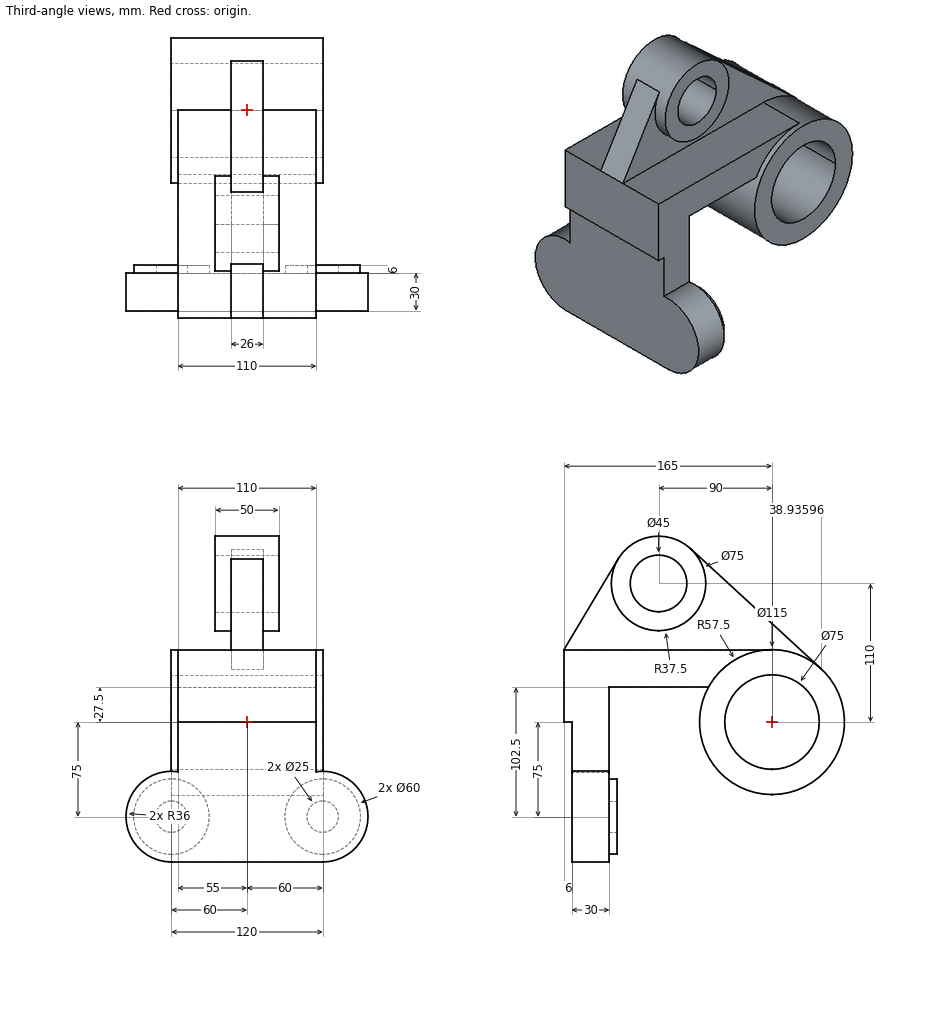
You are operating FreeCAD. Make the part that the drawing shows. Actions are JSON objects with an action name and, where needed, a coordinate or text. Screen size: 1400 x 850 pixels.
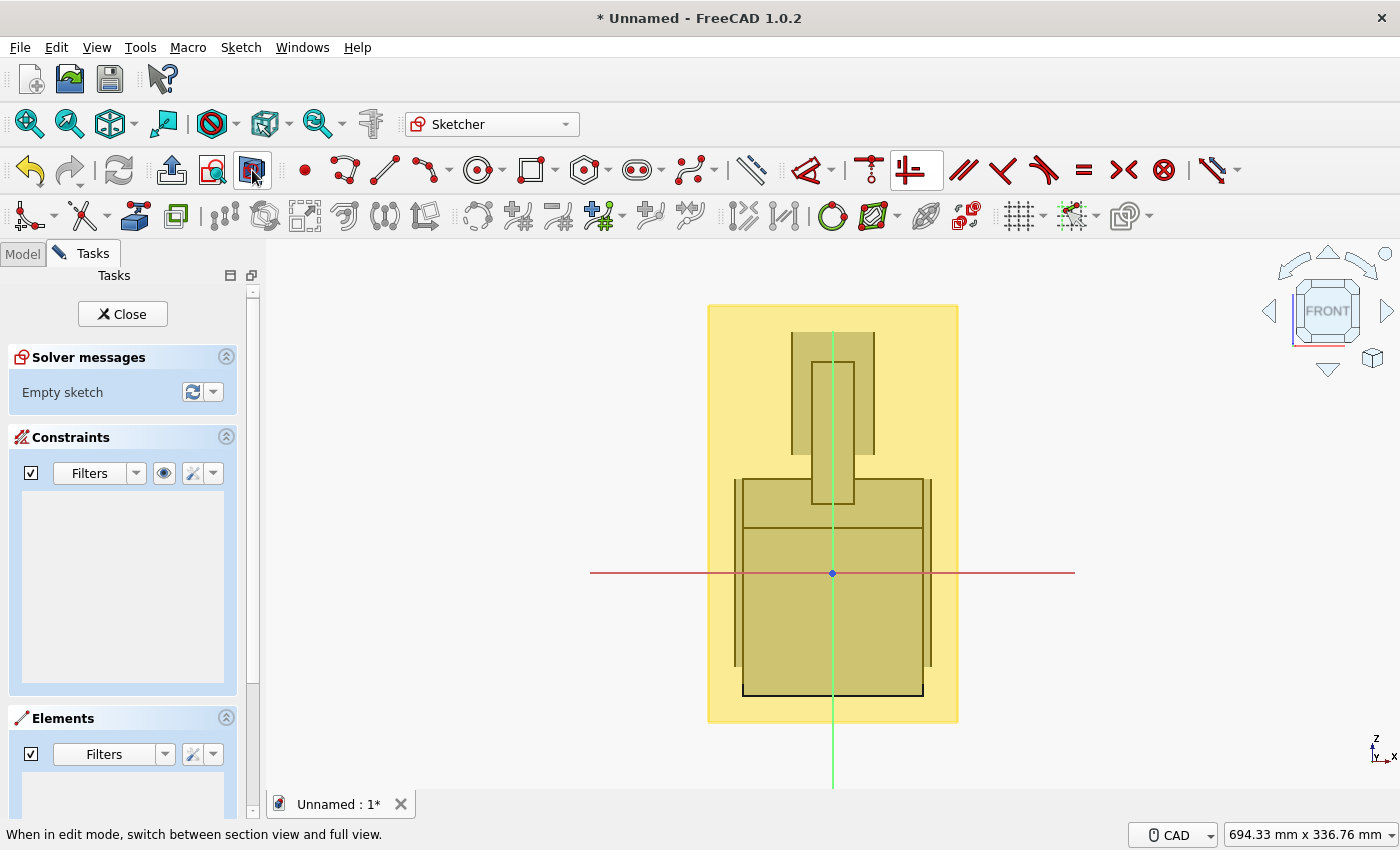
{"action": "scroll", "coordinate": [455, 267], "scroll_direction": "down", "scroll_amount": 1}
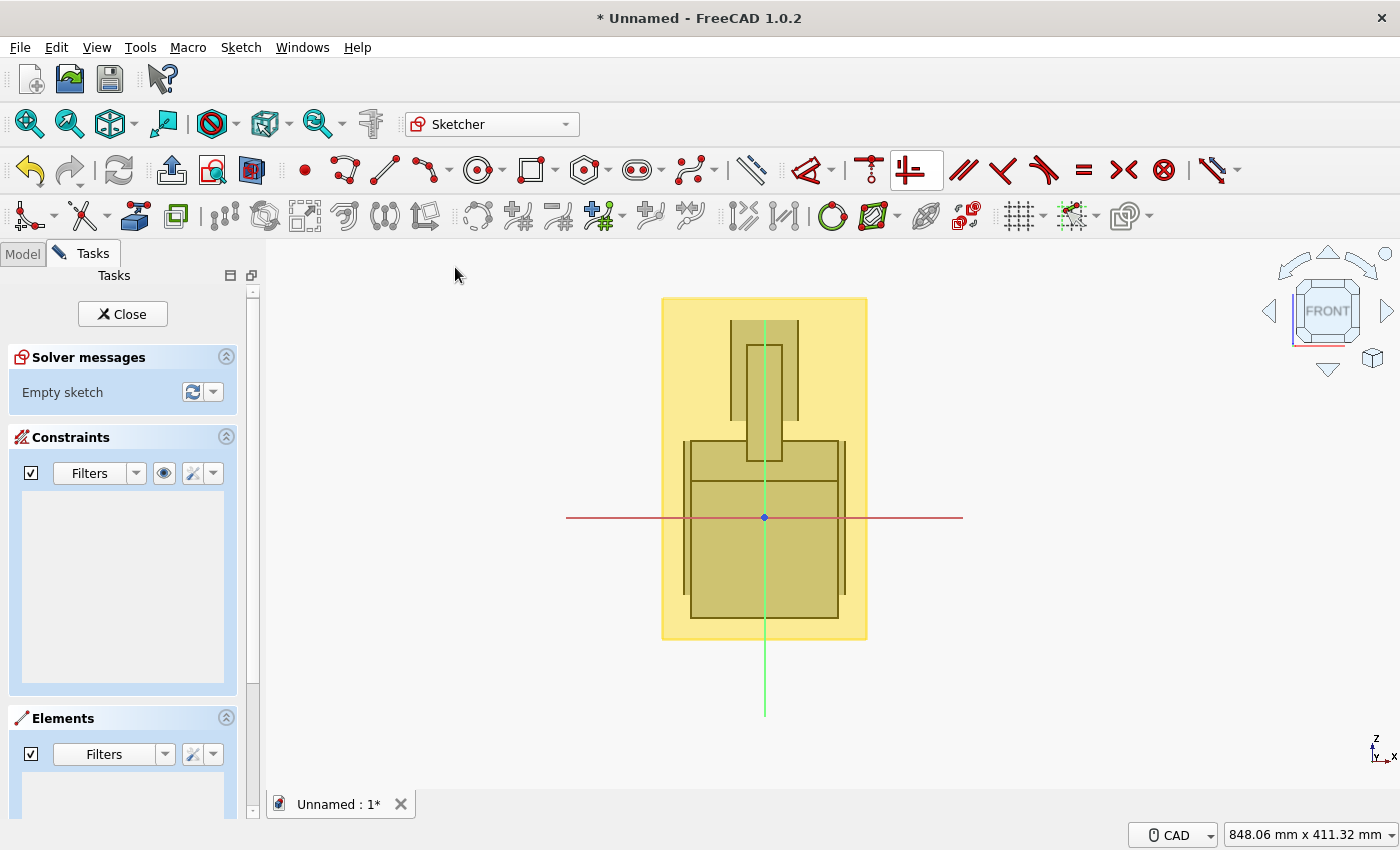
{"action": "scroll", "coordinate": [765, 646], "scroll_direction": "up", "scroll_amount": 3}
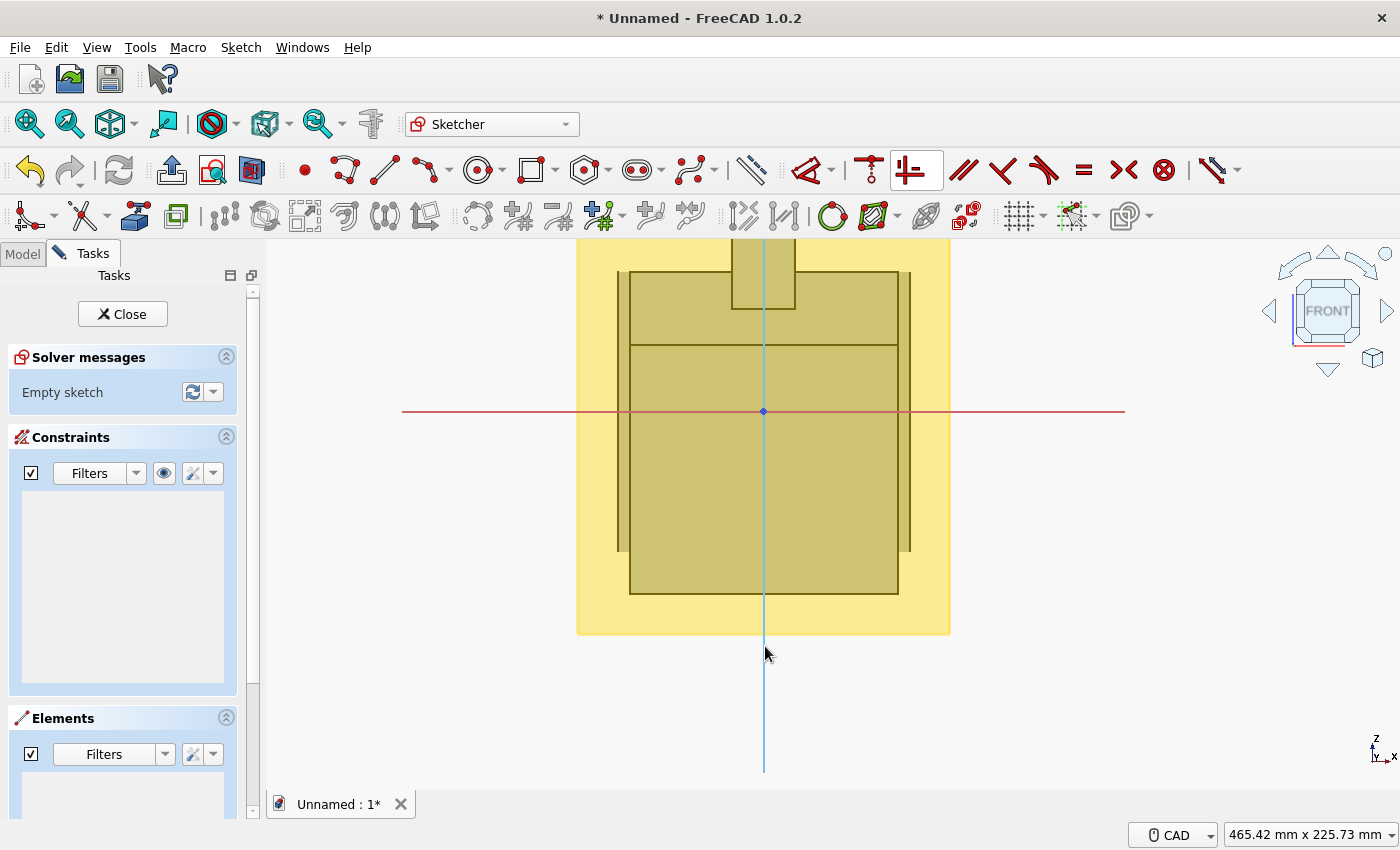
{"action": "left_click", "coordinate": [386, 170]}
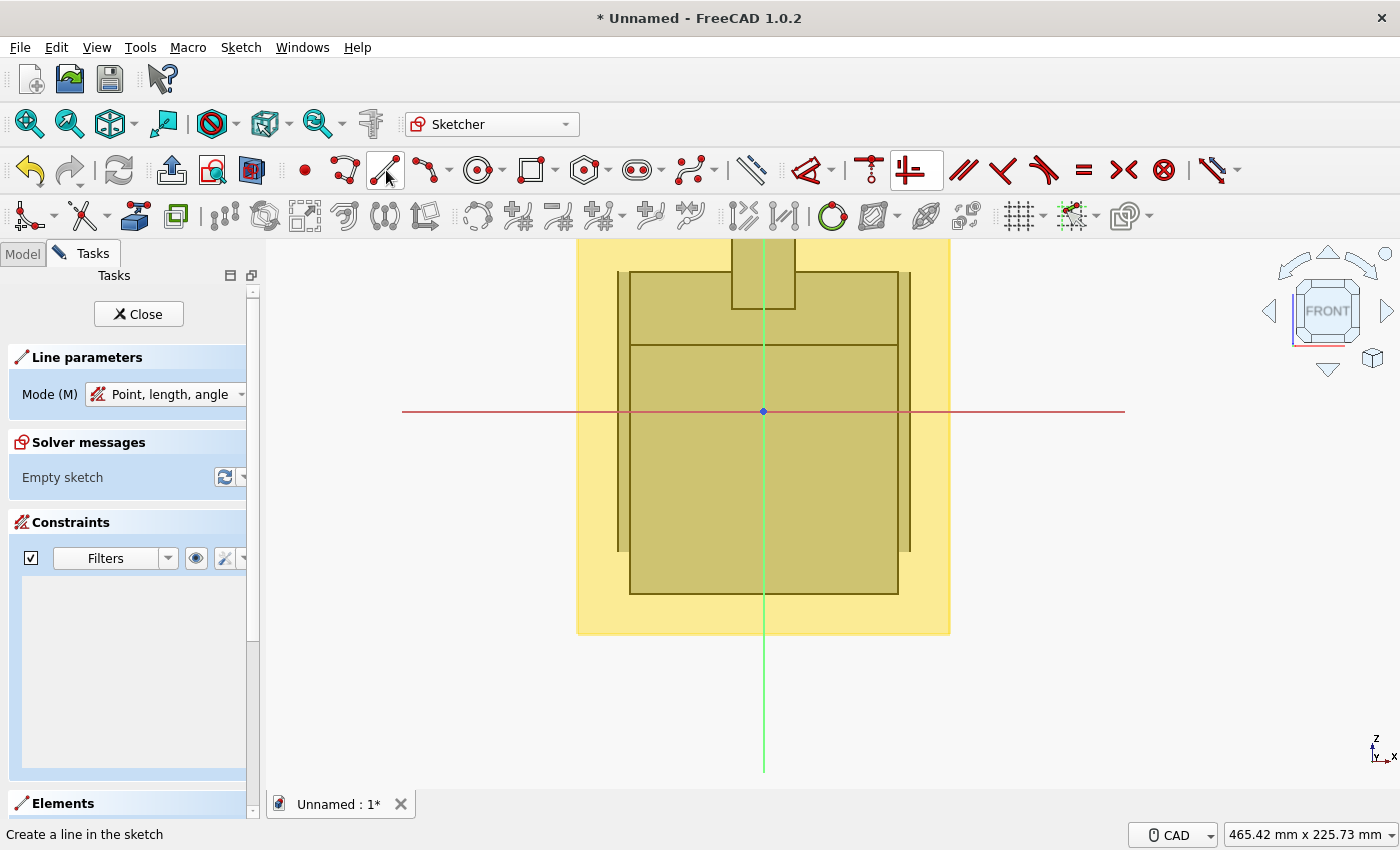
{"action": "left_click", "coordinate": [910, 682]}
{"action": "left_click", "coordinate": [618, 682]}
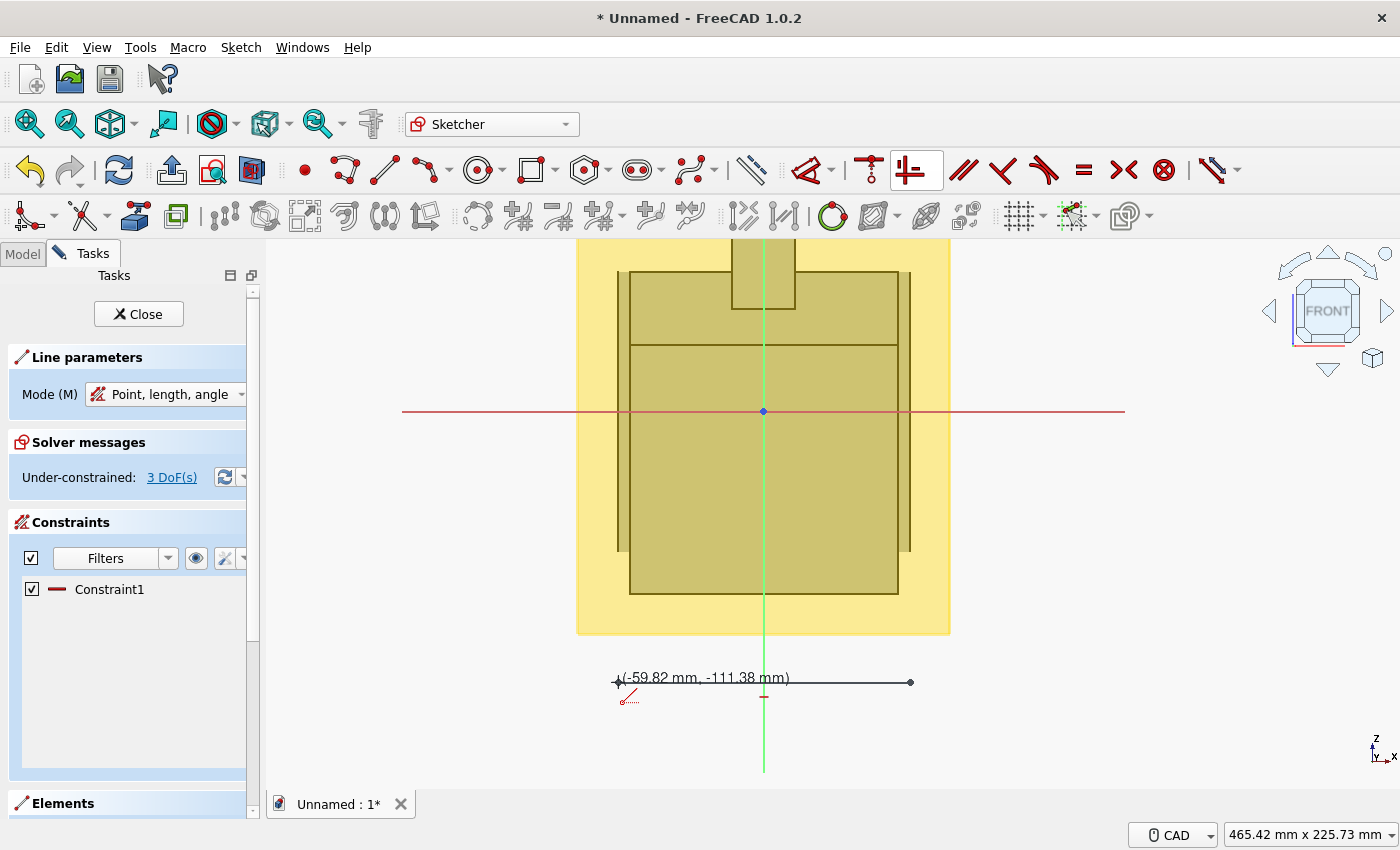
{"action": "left_click", "coordinate": [346, 170]}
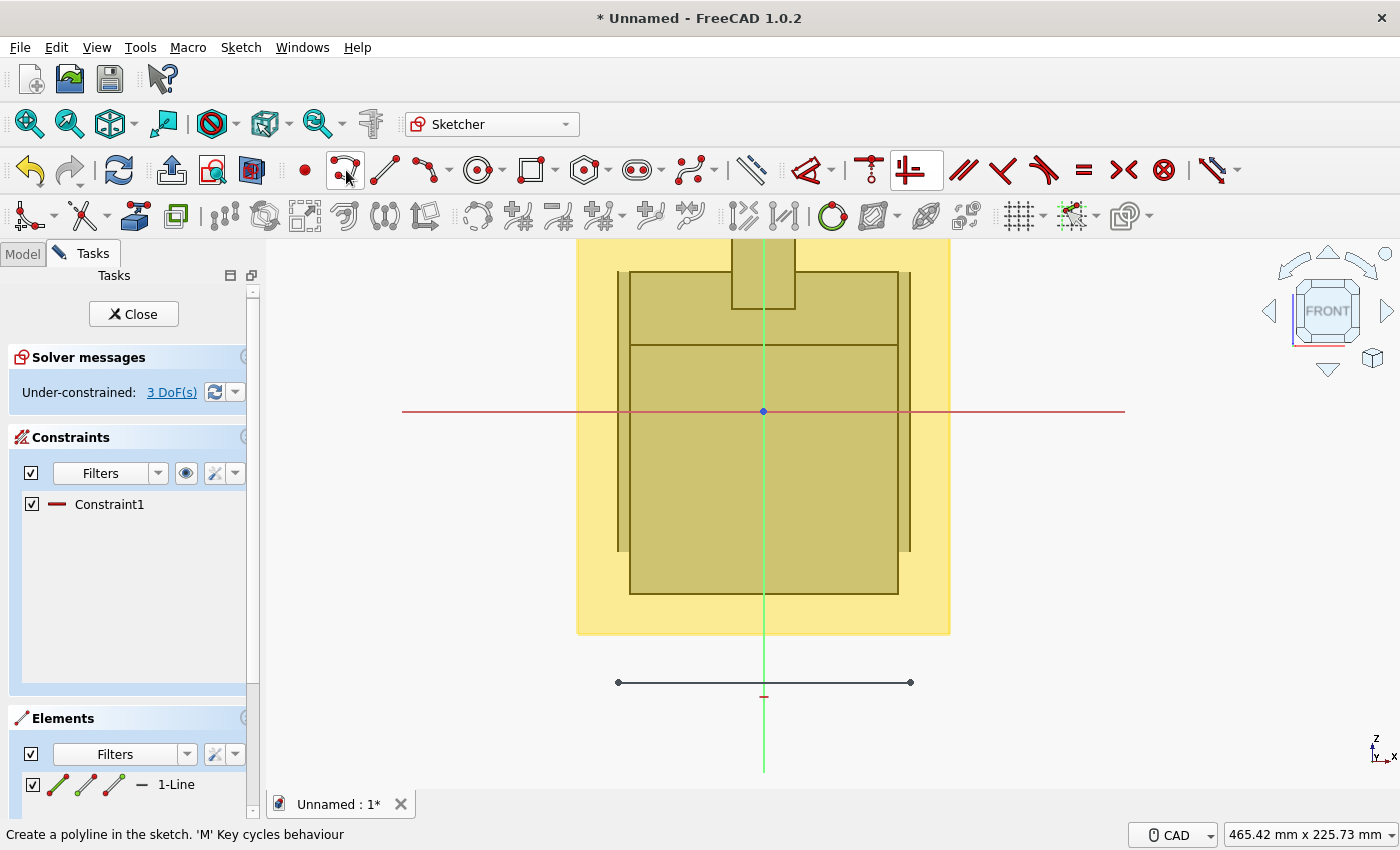
{"action": "left_click", "coordinate": [630, 507]}
{"action": "left_click", "coordinate": [630, 345]}
{"action": "left_click", "coordinate": [898, 345]}
{"action": "left_click", "coordinate": [898, 507]}
{"action": "right_click", "coordinate": [898, 507]}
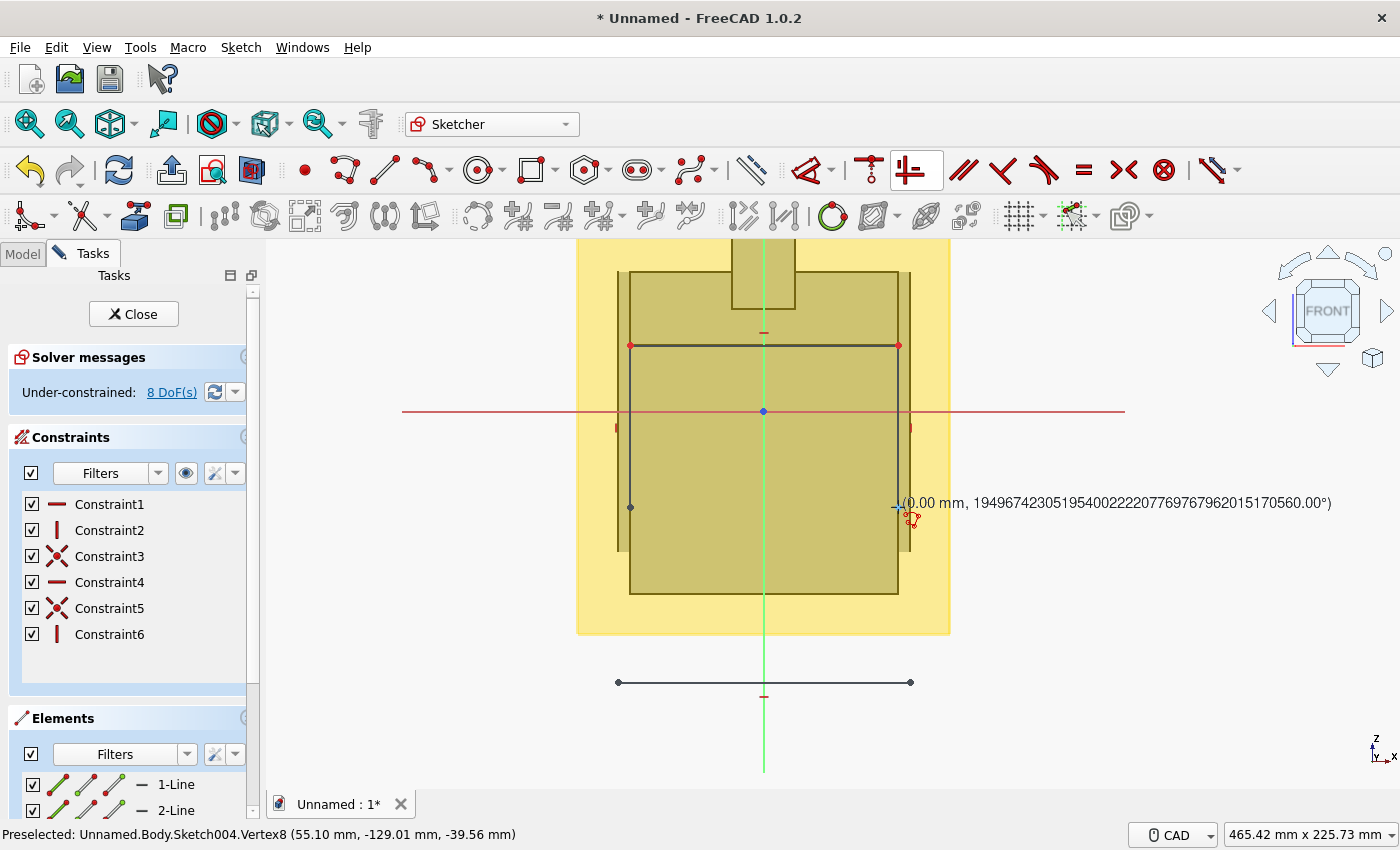
{"action": "left_click", "coordinate": [426, 170]}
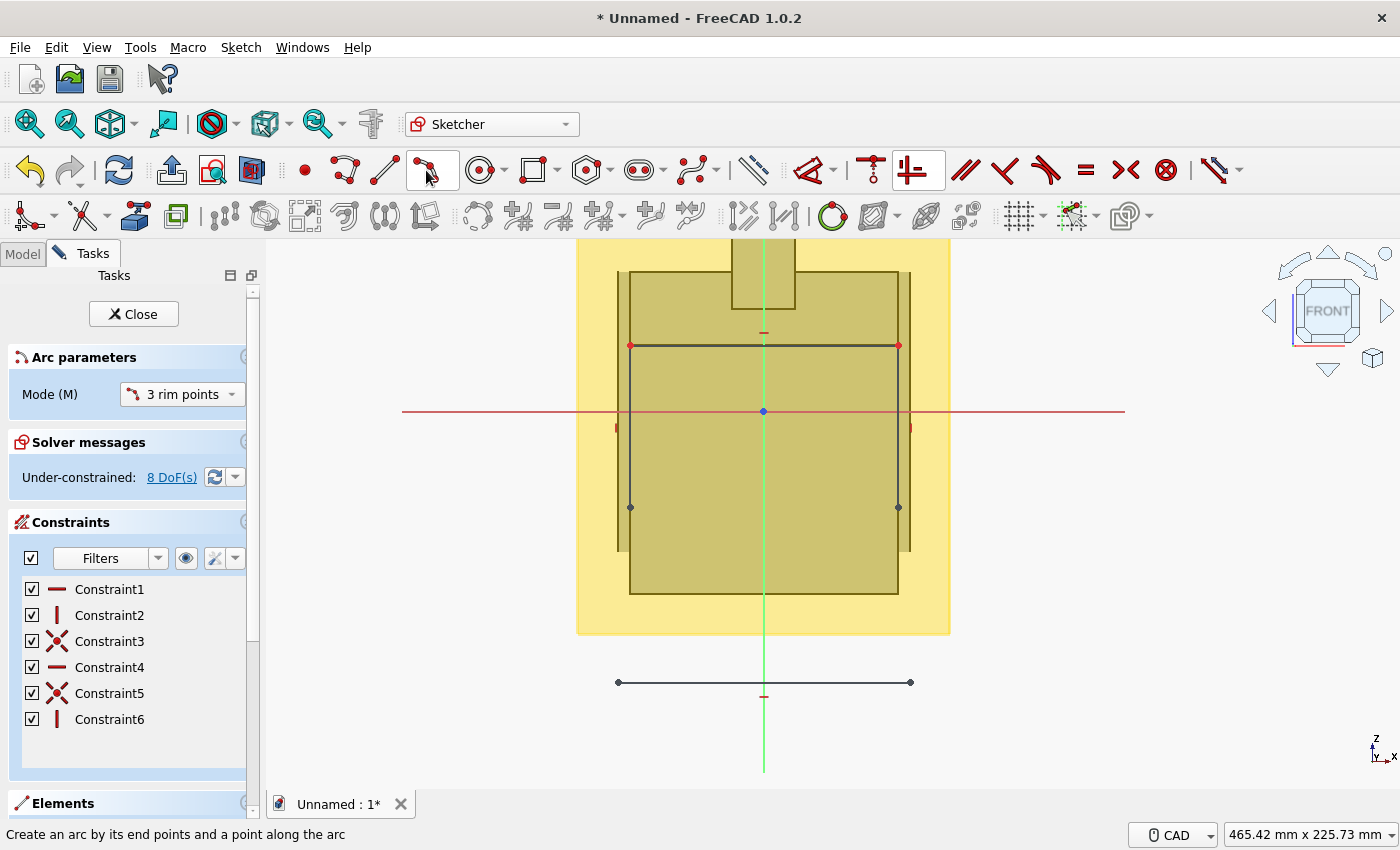
{"action": "left_click", "coordinate": [618, 683]}
{"action": "left_click", "coordinate": [630, 508]}
{"action": "left_click", "coordinate": [530, 588]}